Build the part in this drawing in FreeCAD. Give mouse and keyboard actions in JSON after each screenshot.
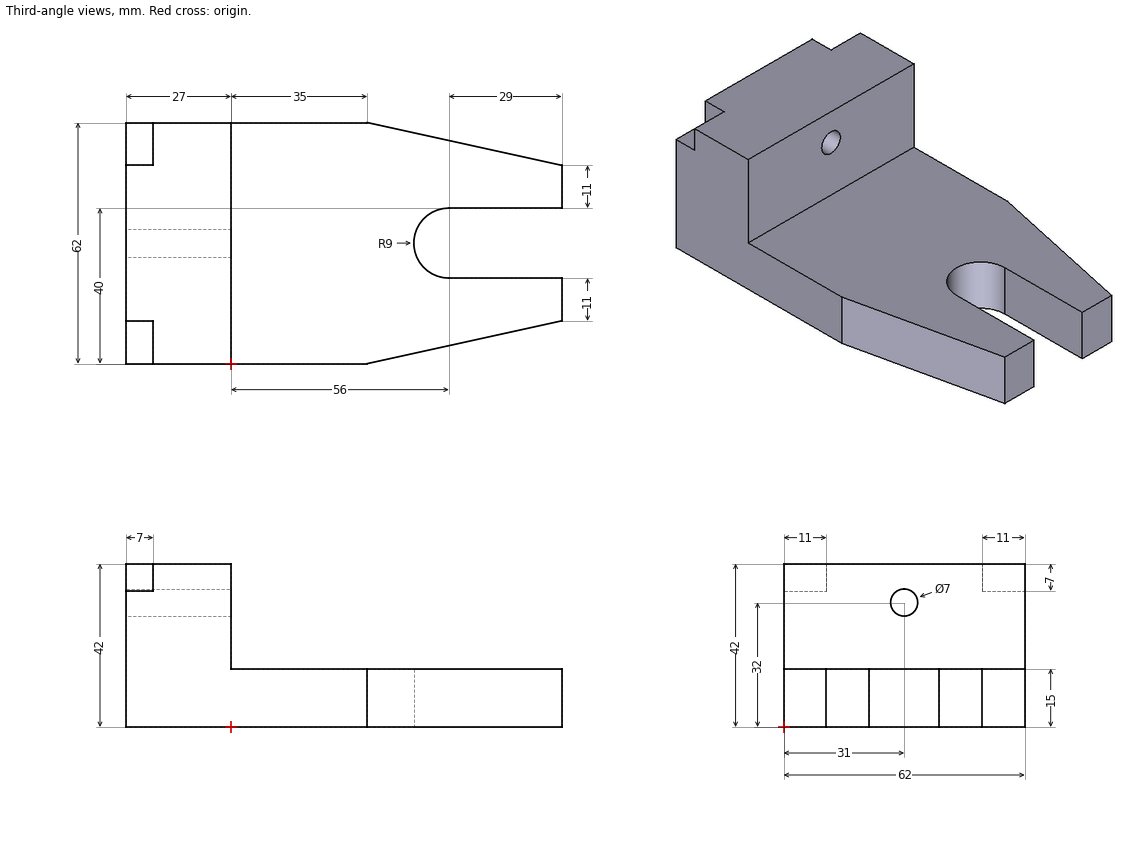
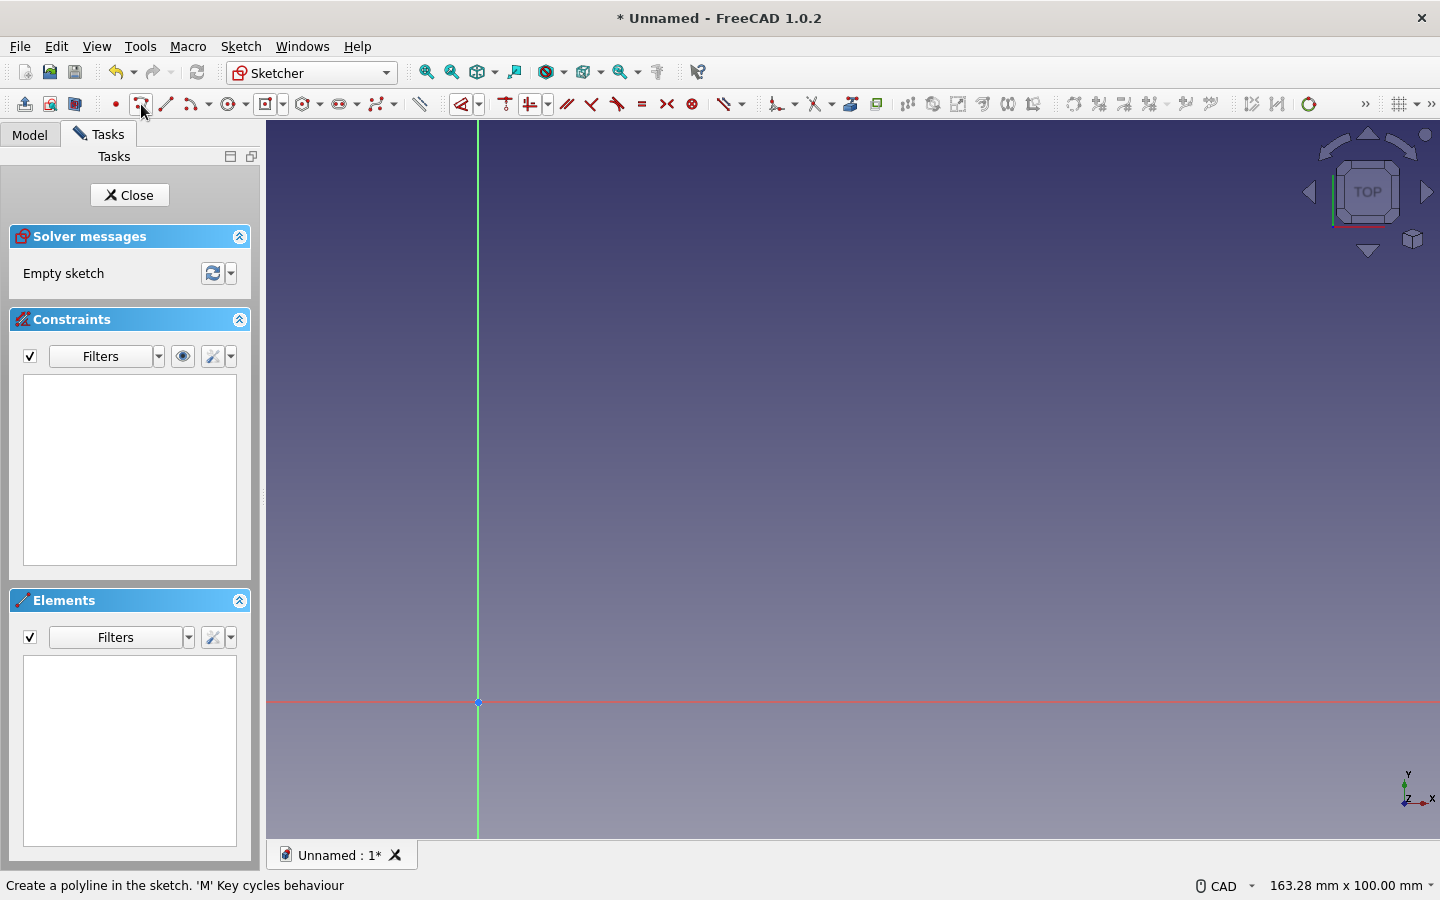
{"action": "left_click", "coordinate": [881, 415]}
{"action": "left_click", "coordinate": [1090, 415]}
{"action": "left_click", "coordinate": [1090, 335]}
{"action": "left_click", "coordinate": [730, 256]}
{"action": "left_click", "coordinate": [478, 256]}
{"action": "left_click", "coordinate": [478, 702]}
{"action": "left_click", "coordinate": [730, 693]}
{"action": "left_click", "coordinate": [1090, 623]}
{"action": "left_click", "coordinate": [1090, 544]}
{"action": "left_click", "coordinate": [881, 544]}
{"action": "right_click", "coordinate": [881, 544]}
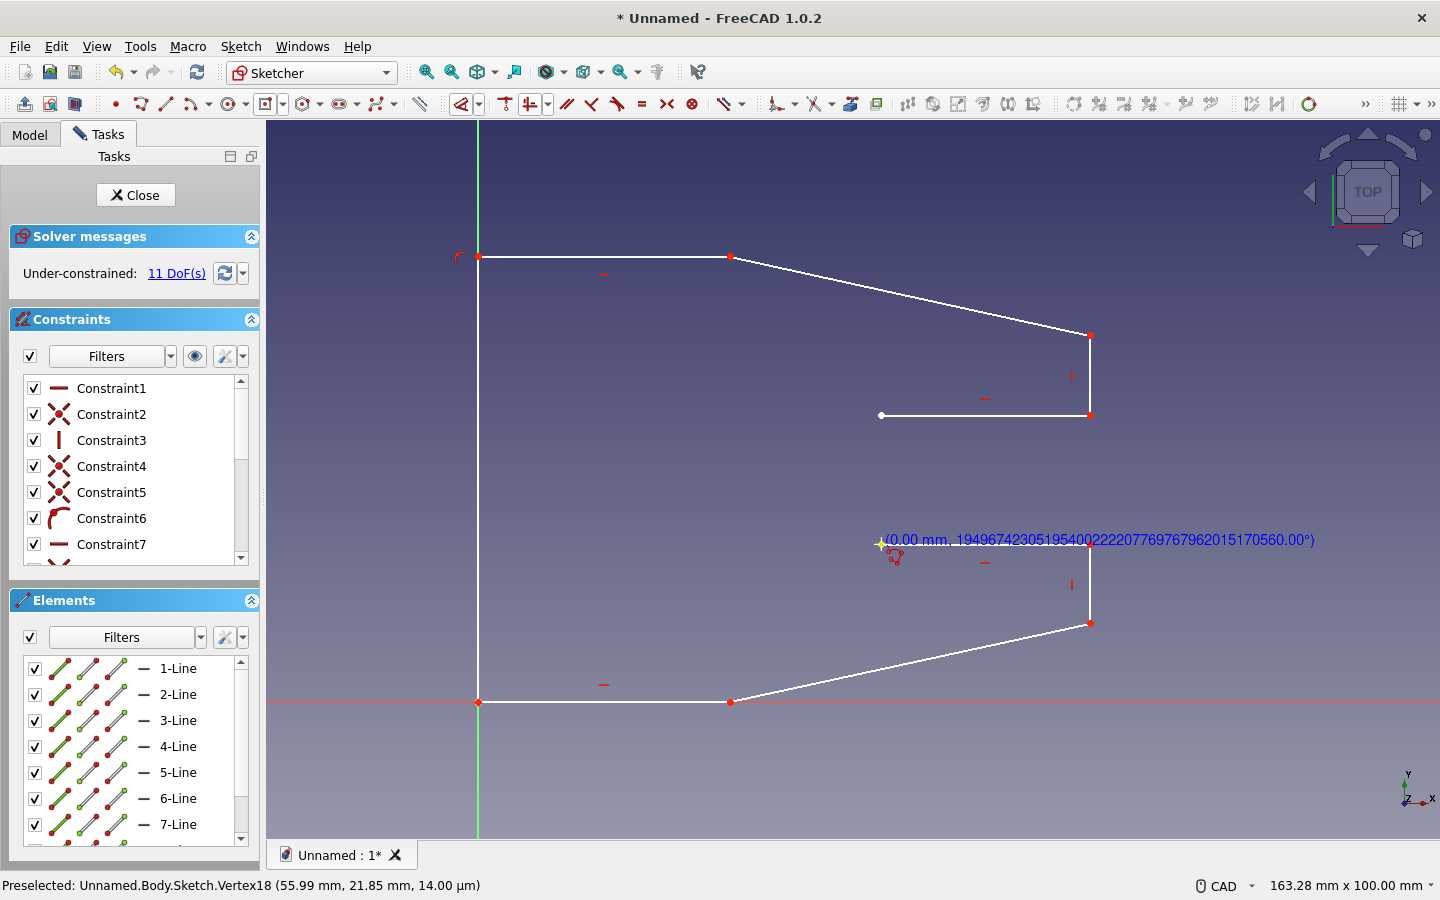
{"action": "left_click", "coordinate": [208, 104]}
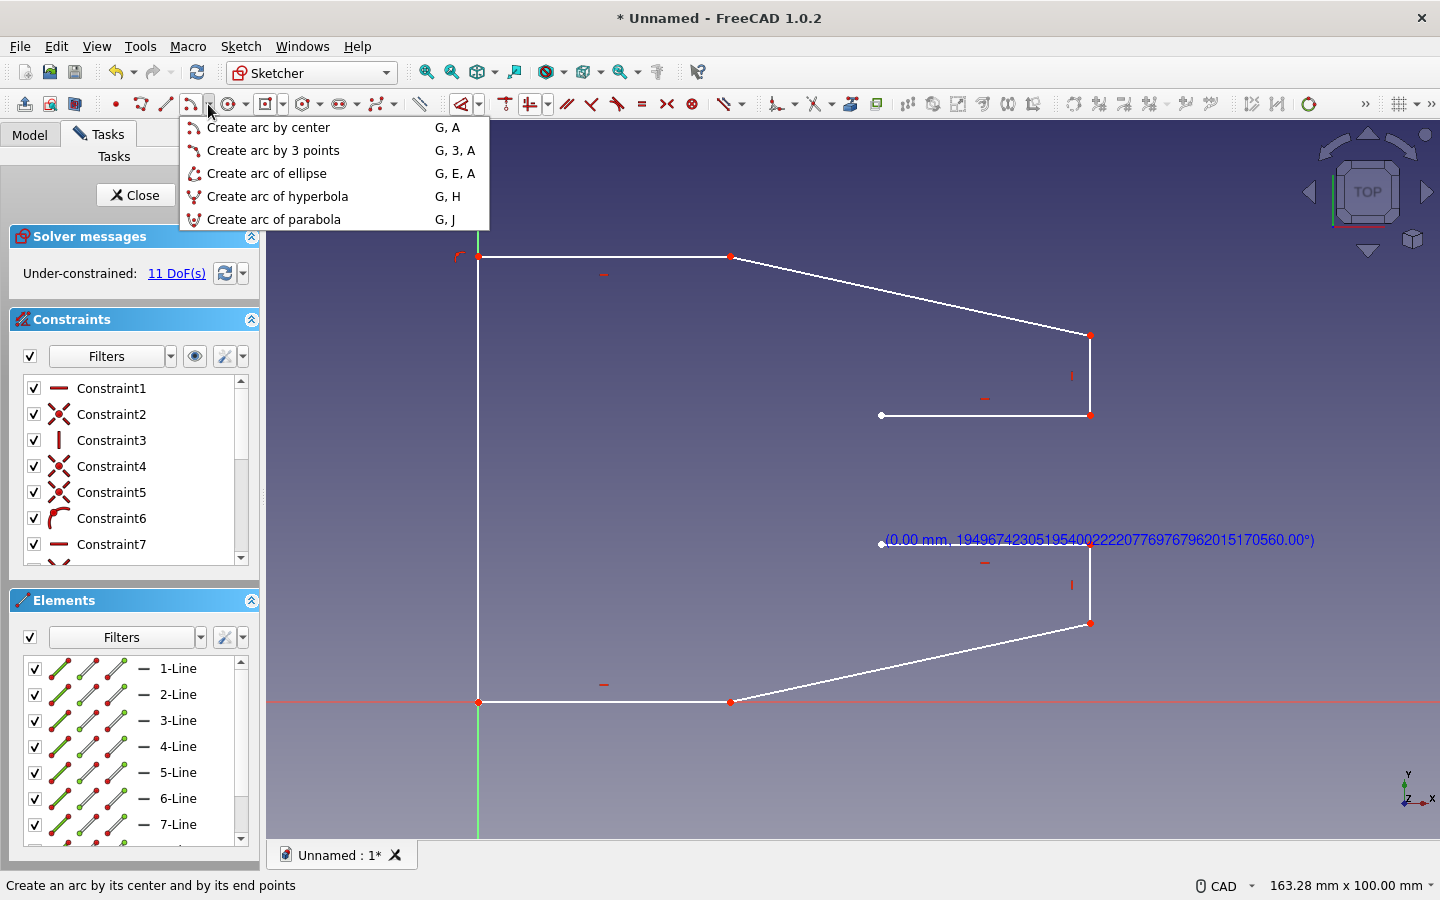
{"action": "left_click", "coordinate": [334, 150]}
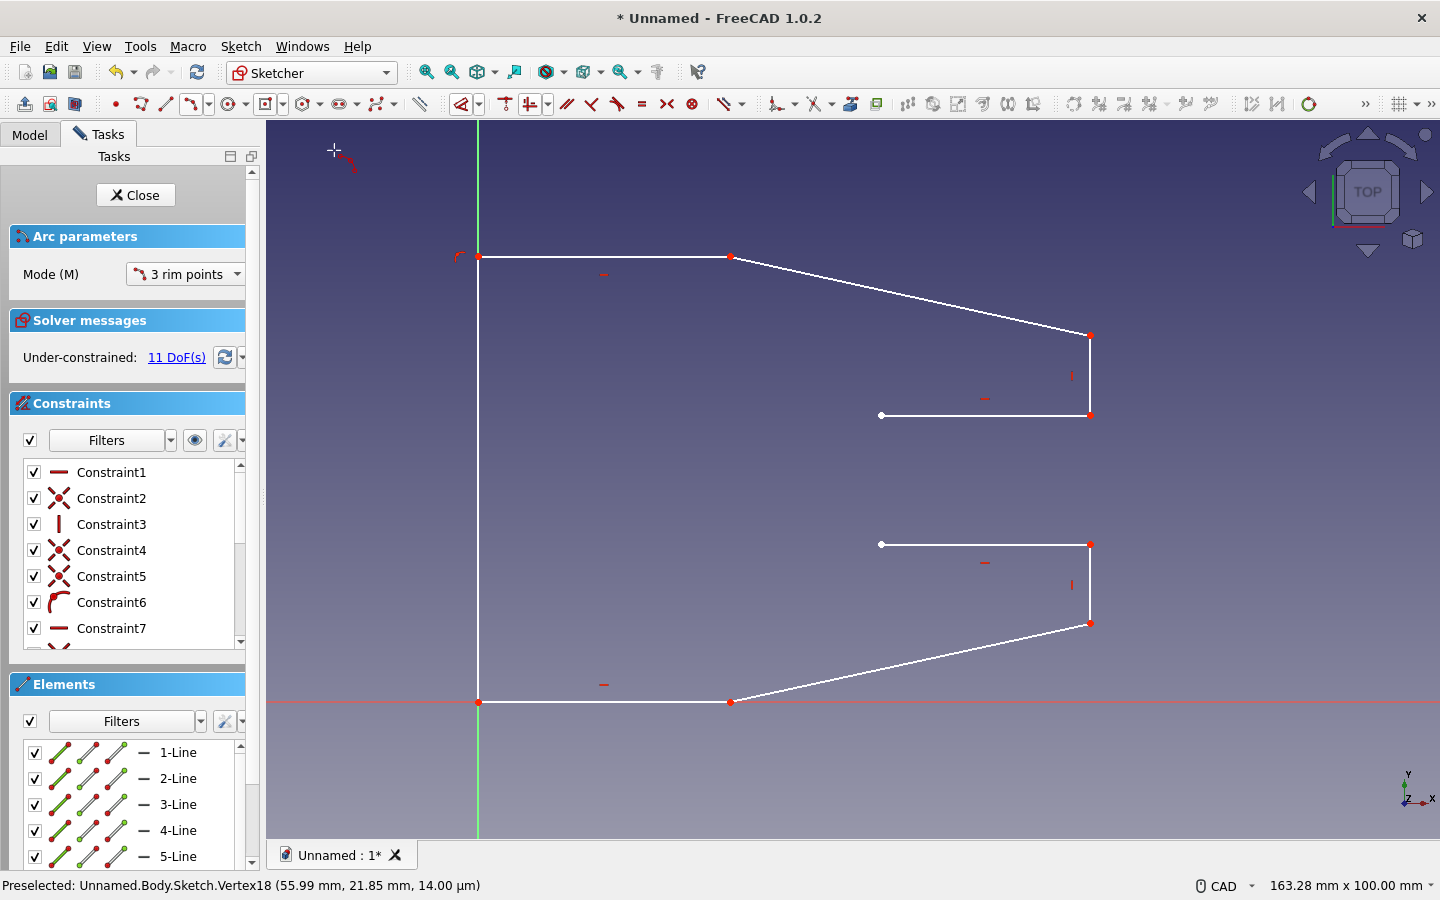
{"action": "left_click", "coordinate": [881, 545]}
{"action": "left_click", "coordinate": [881, 416]}
{"action": "left_click", "coordinate": [816, 479]}
{"action": "key", "text": "Escape"}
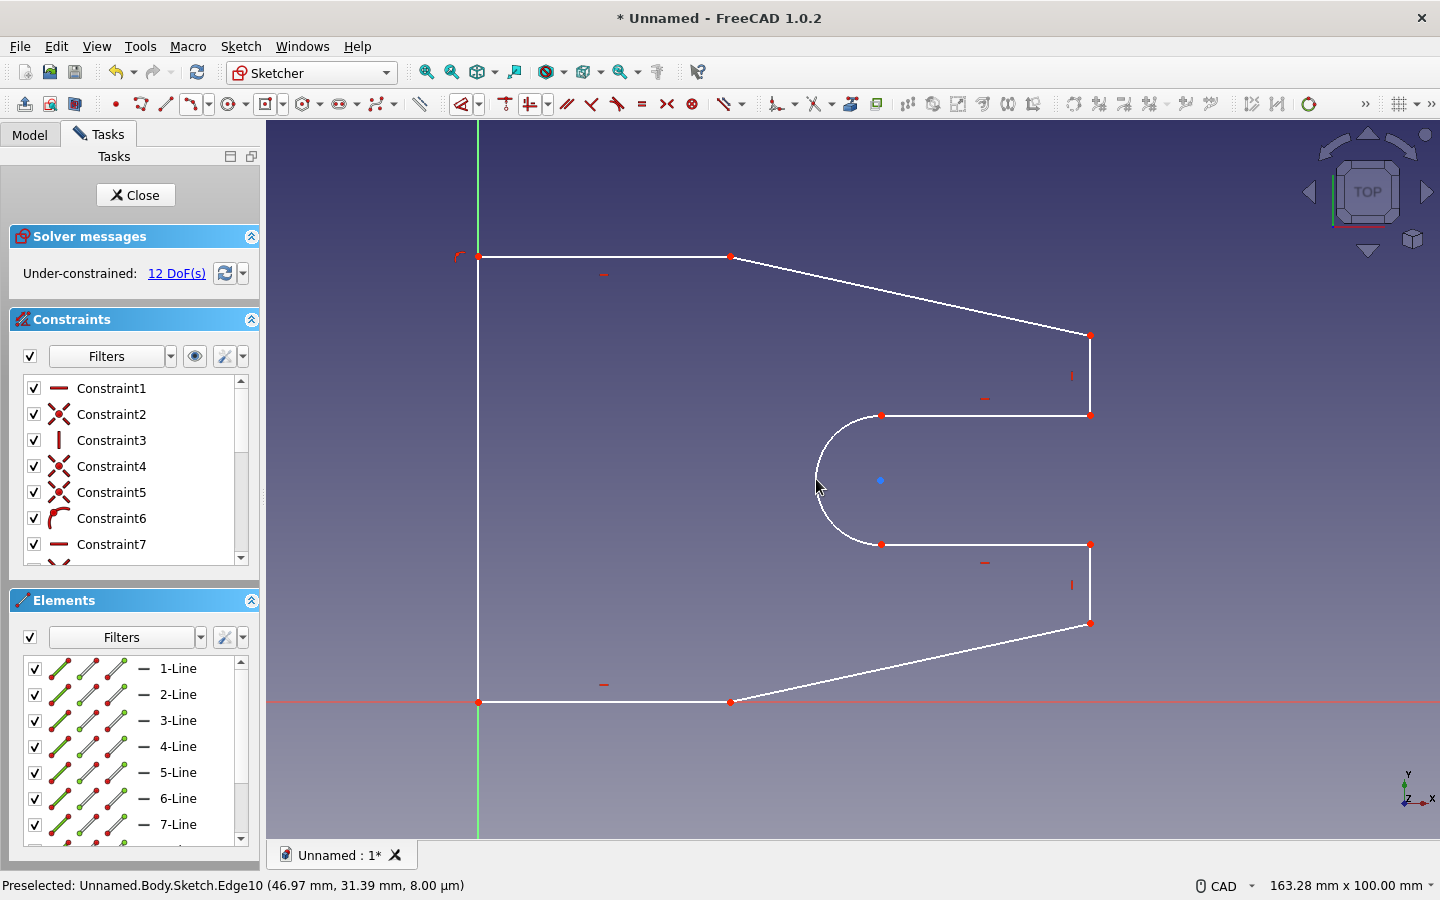
{"action": "left_click", "coordinate": [944, 416]}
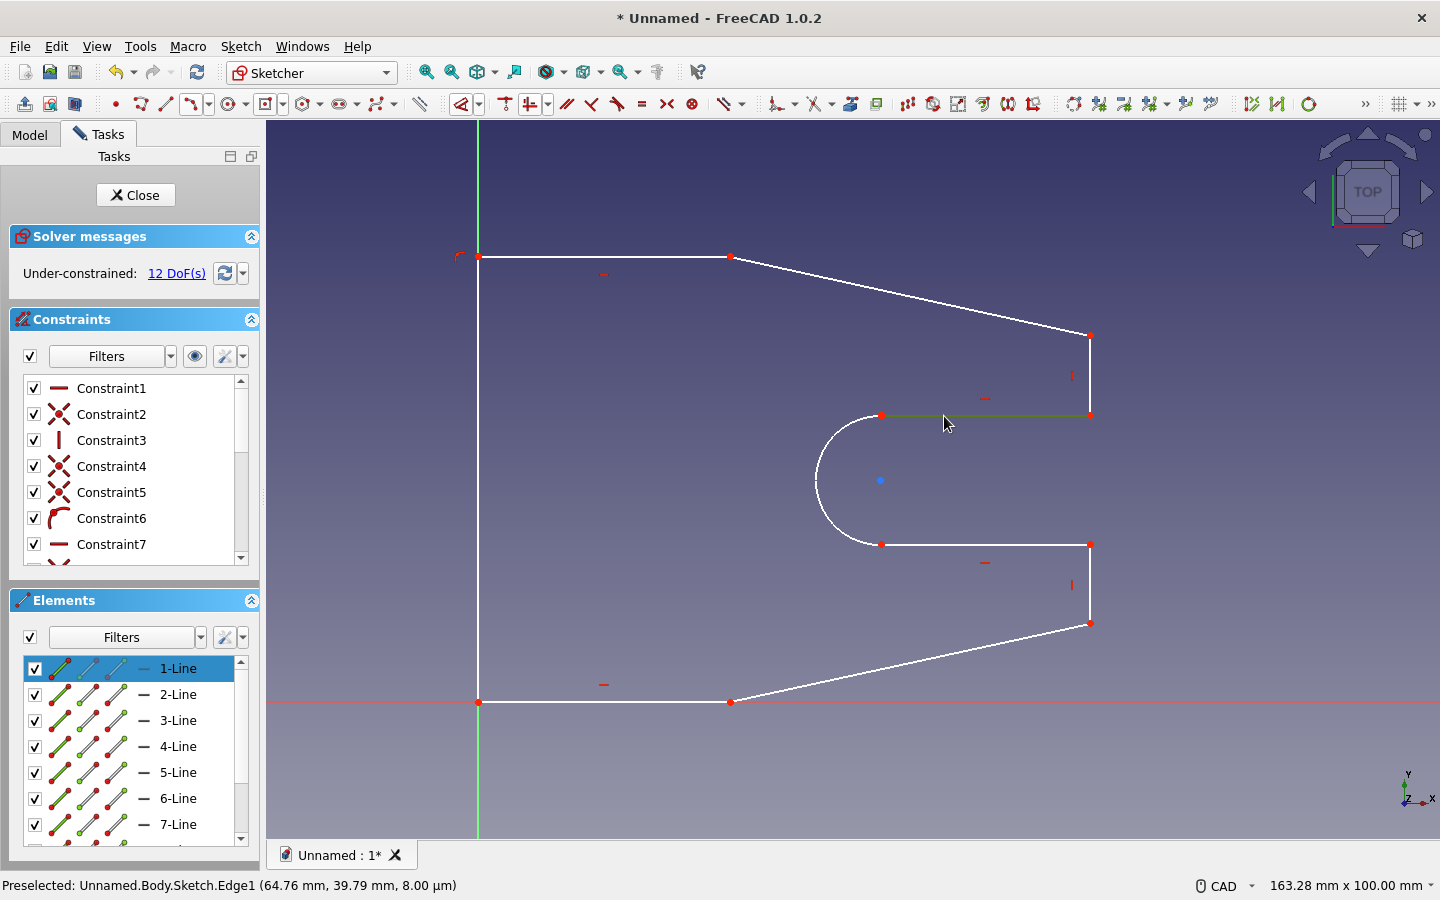
{"action": "left_click", "coordinate": [828, 442]}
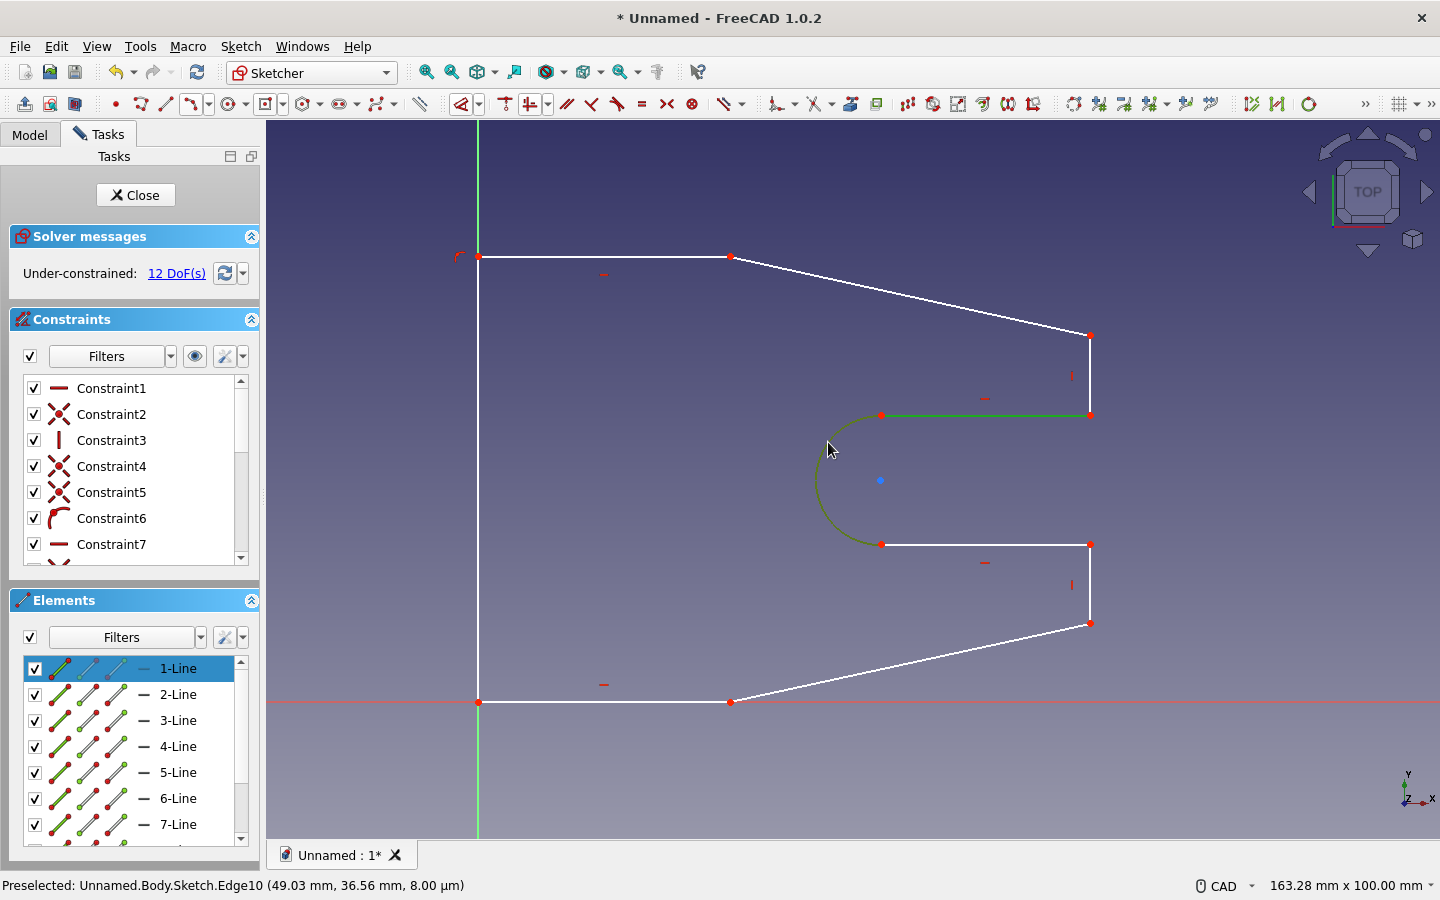
{"action": "left_click", "coordinate": [617, 104]}